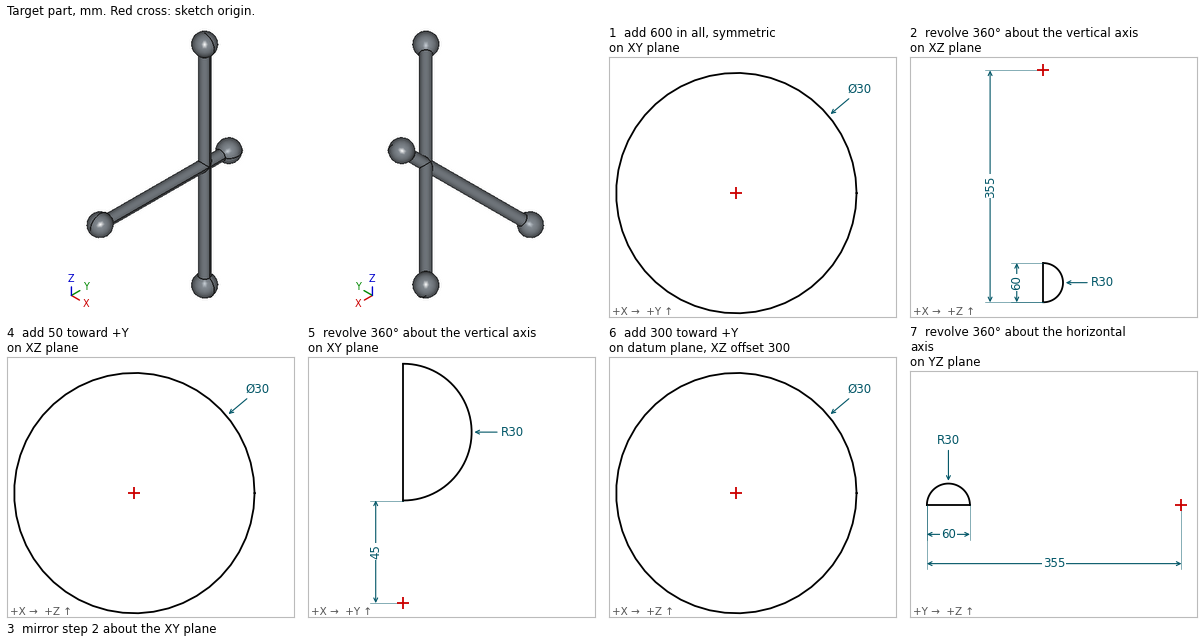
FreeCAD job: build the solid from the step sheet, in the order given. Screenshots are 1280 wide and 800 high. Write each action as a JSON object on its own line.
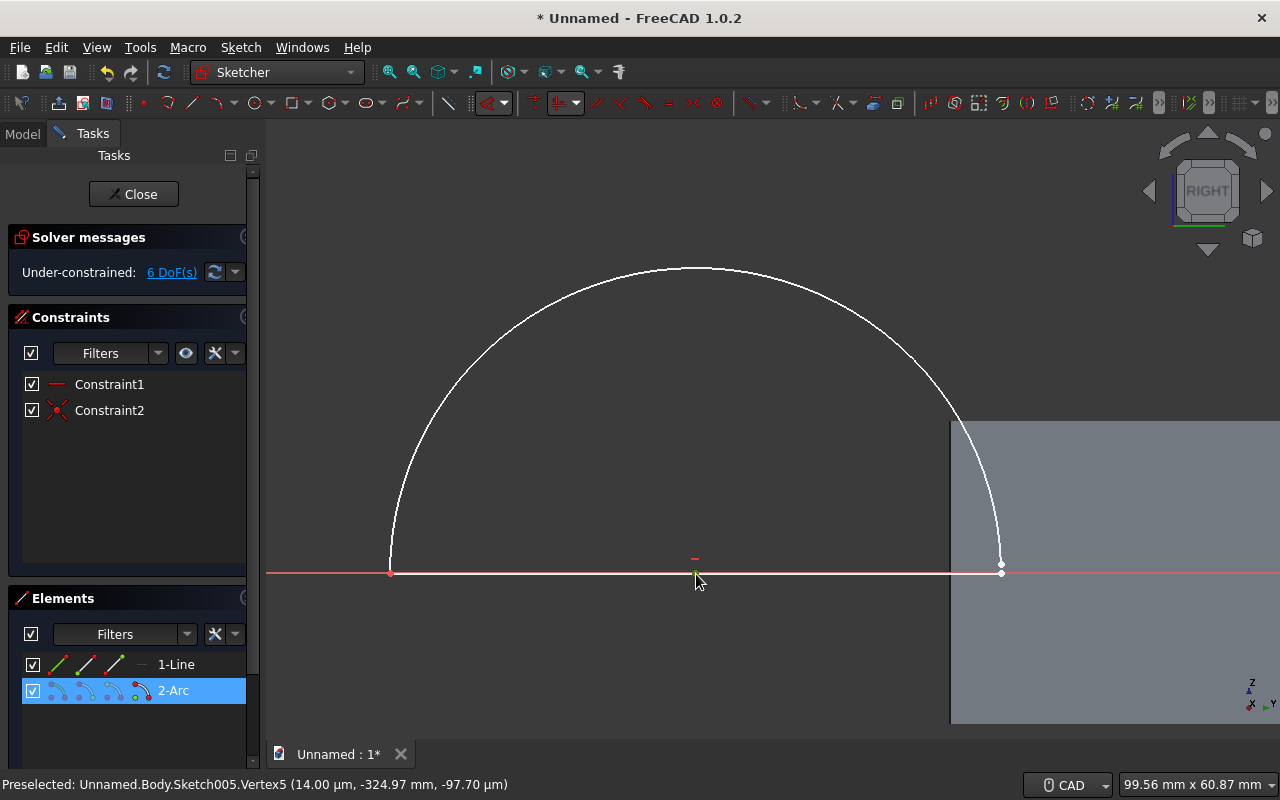
{"action": "left_click", "coordinate": [353, 573]}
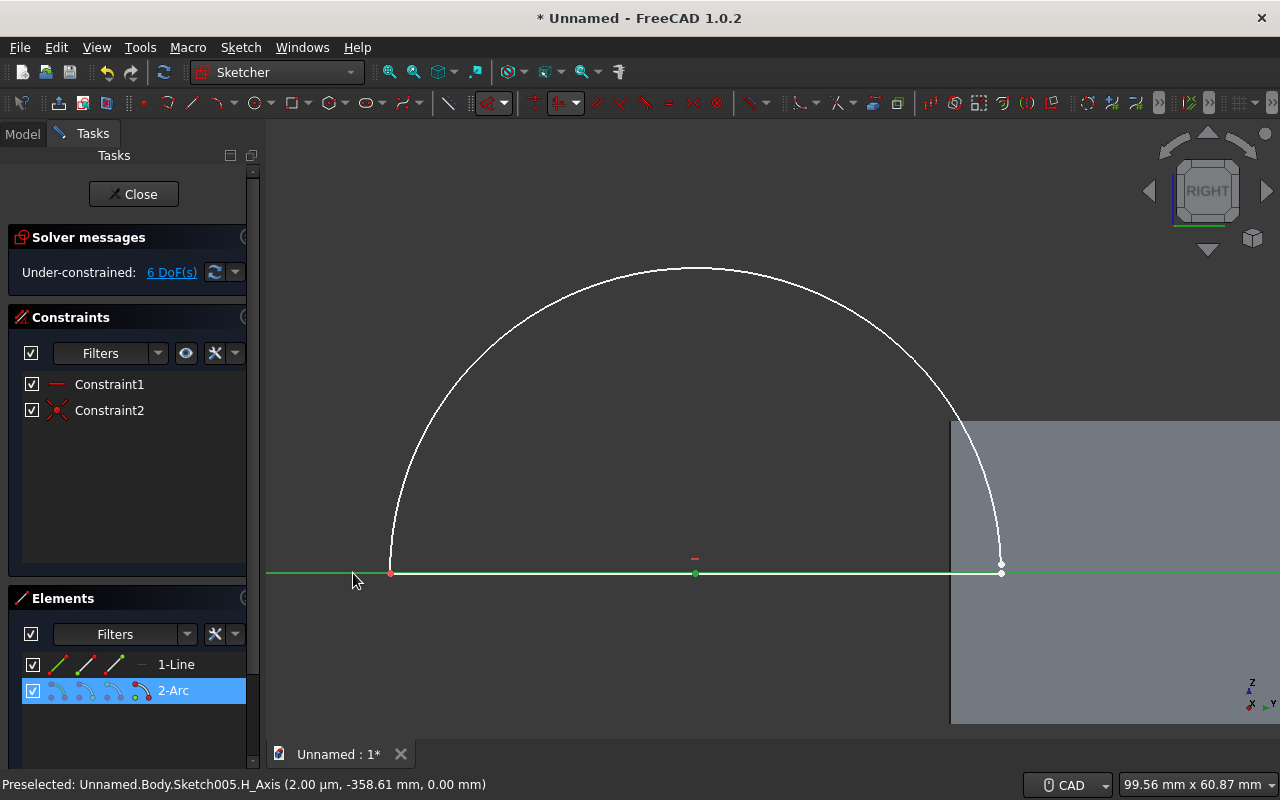
{"action": "left_click", "coordinate": [534, 104]}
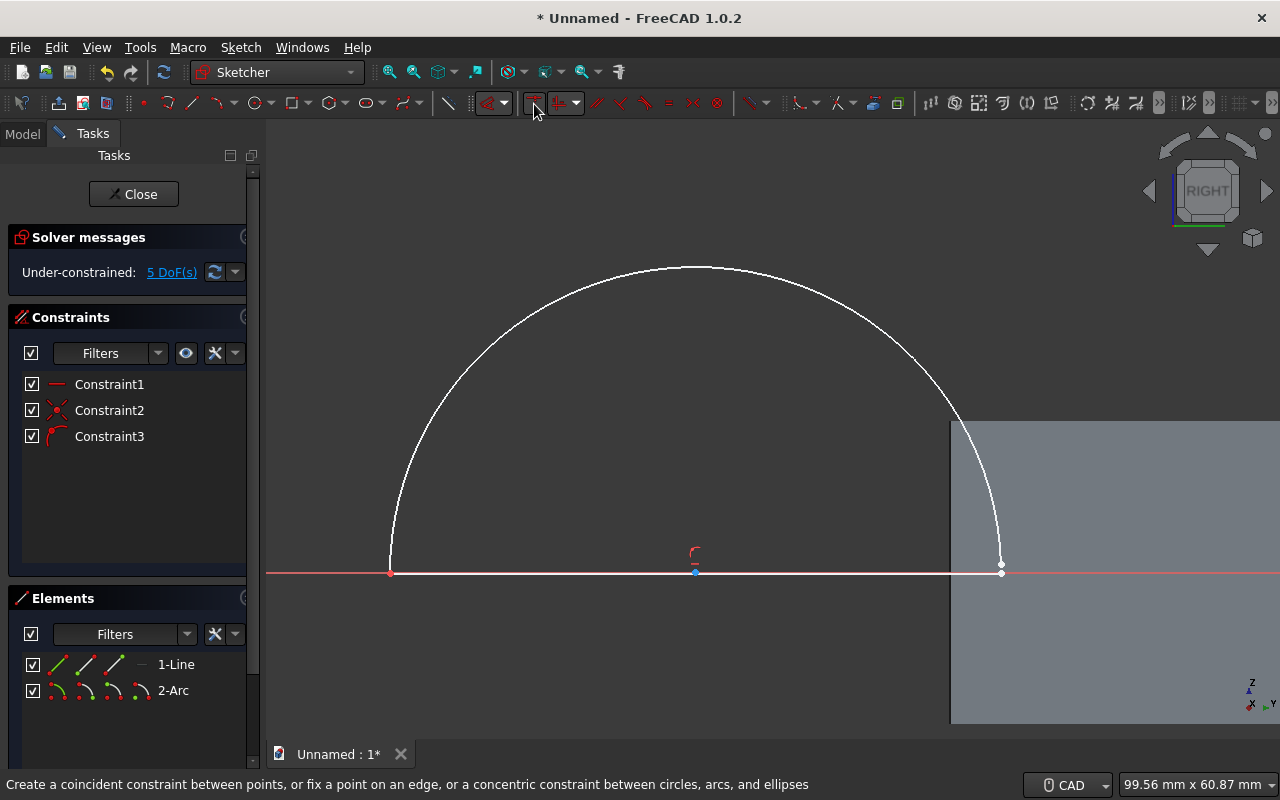
{"action": "left_click", "coordinate": [870, 322]}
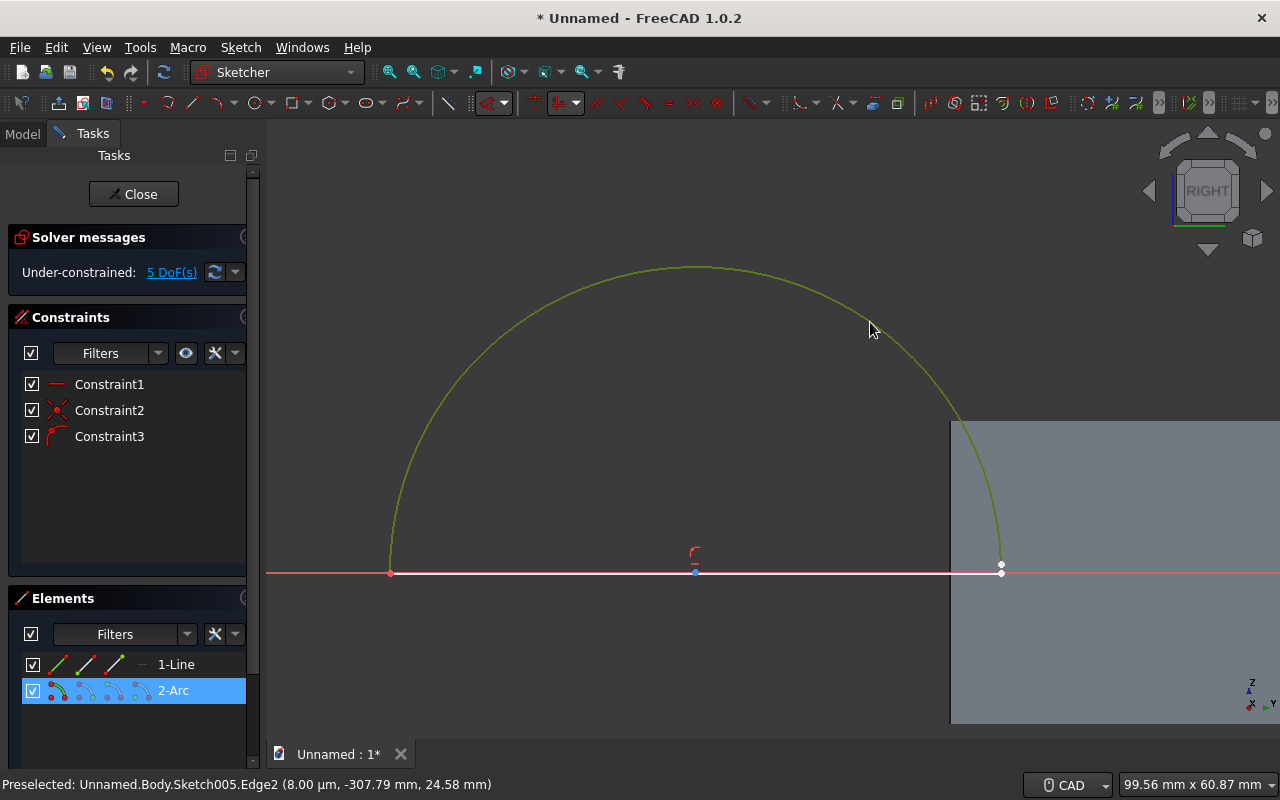
{"action": "key", "text": "k r"}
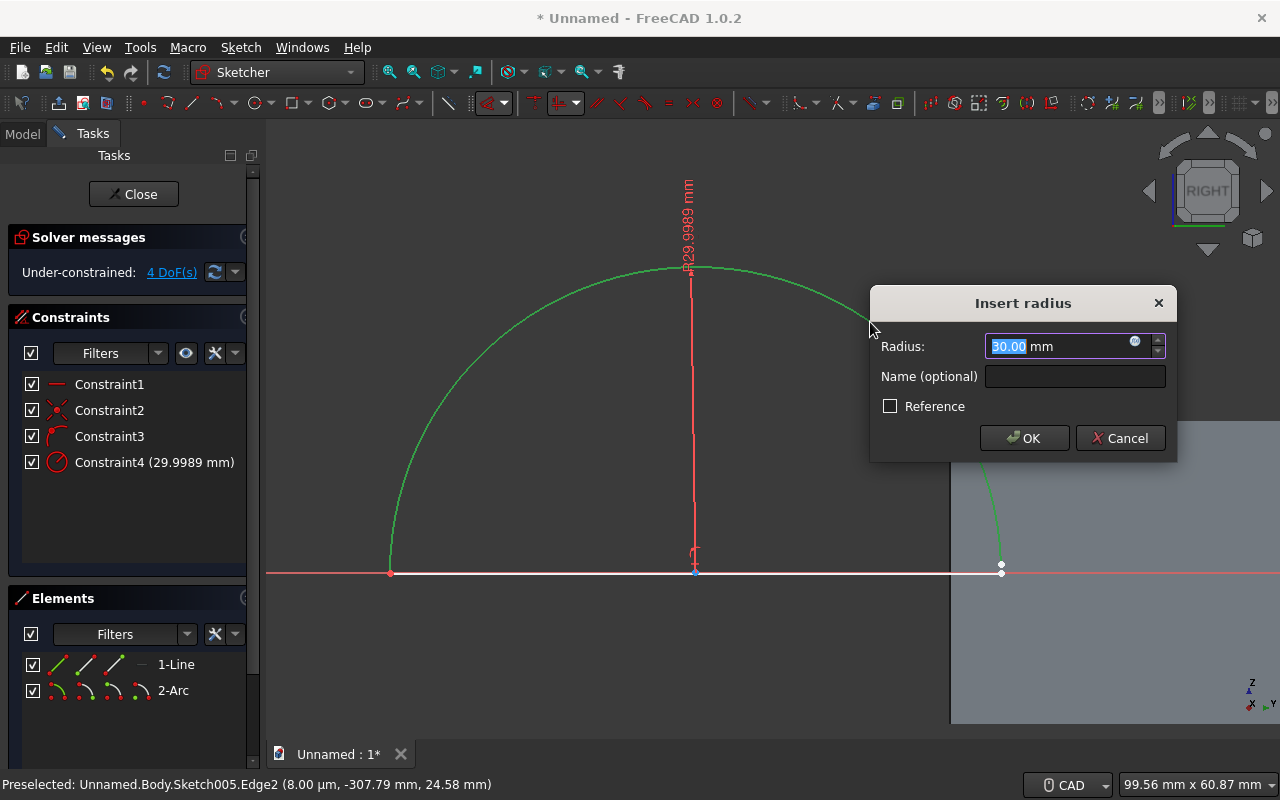
{"action": "type", "text": "30"}
{"action": "key", "text": "Return"}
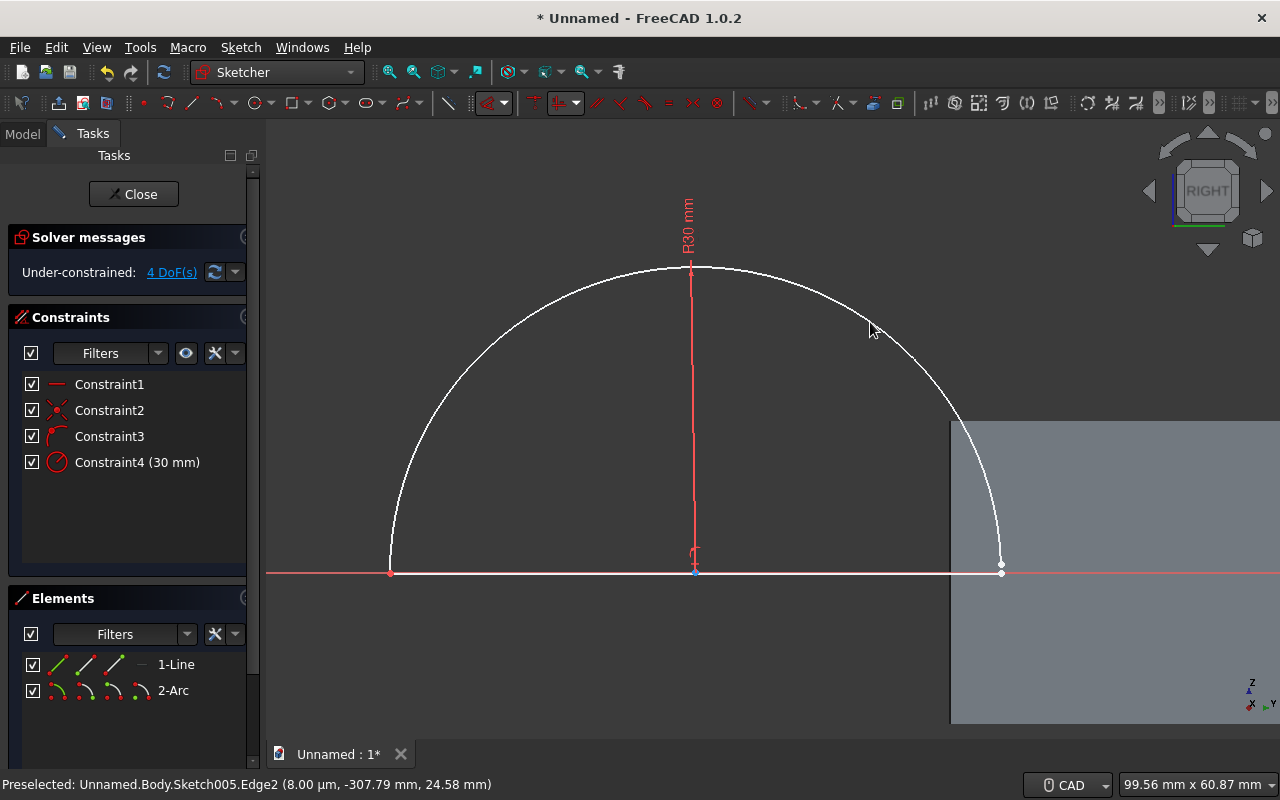
{"action": "left_click", "coordinate": [390, 574]}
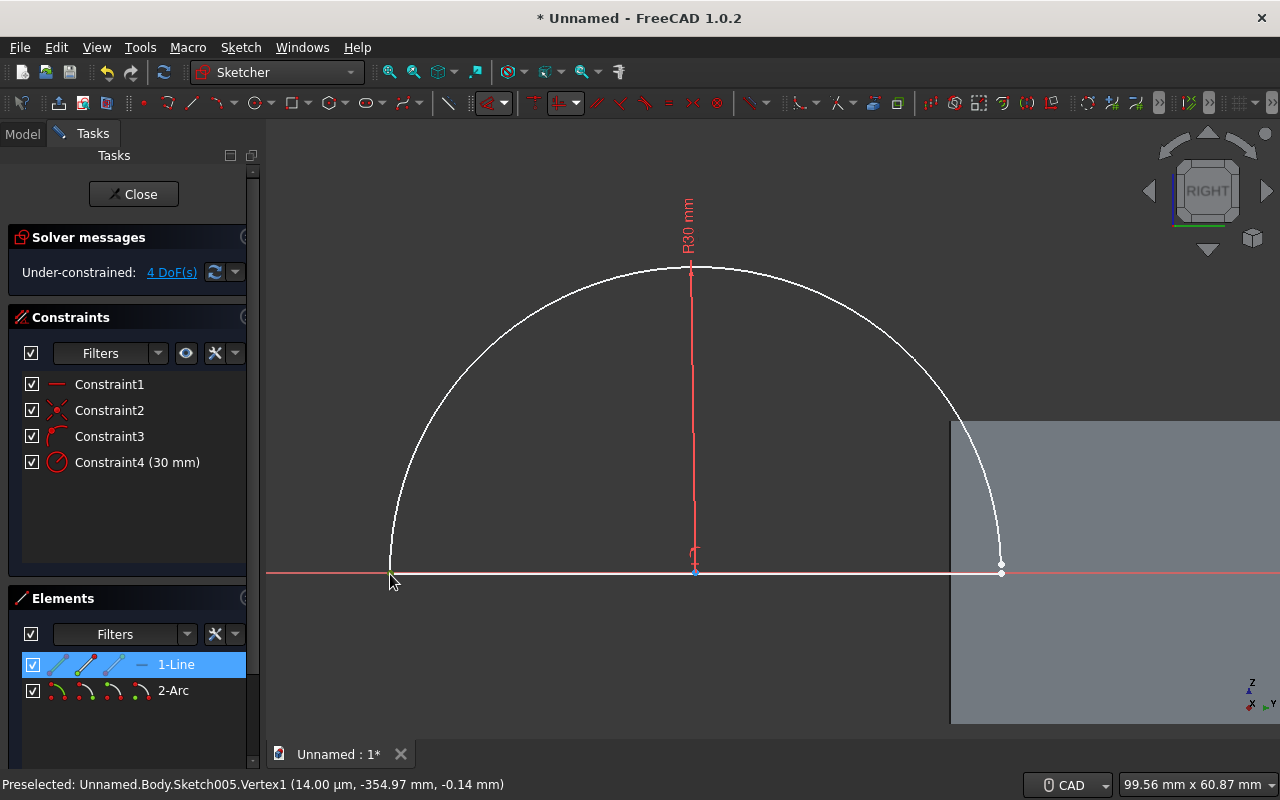
{"action": "left_click", "coordinate": [353, 573]}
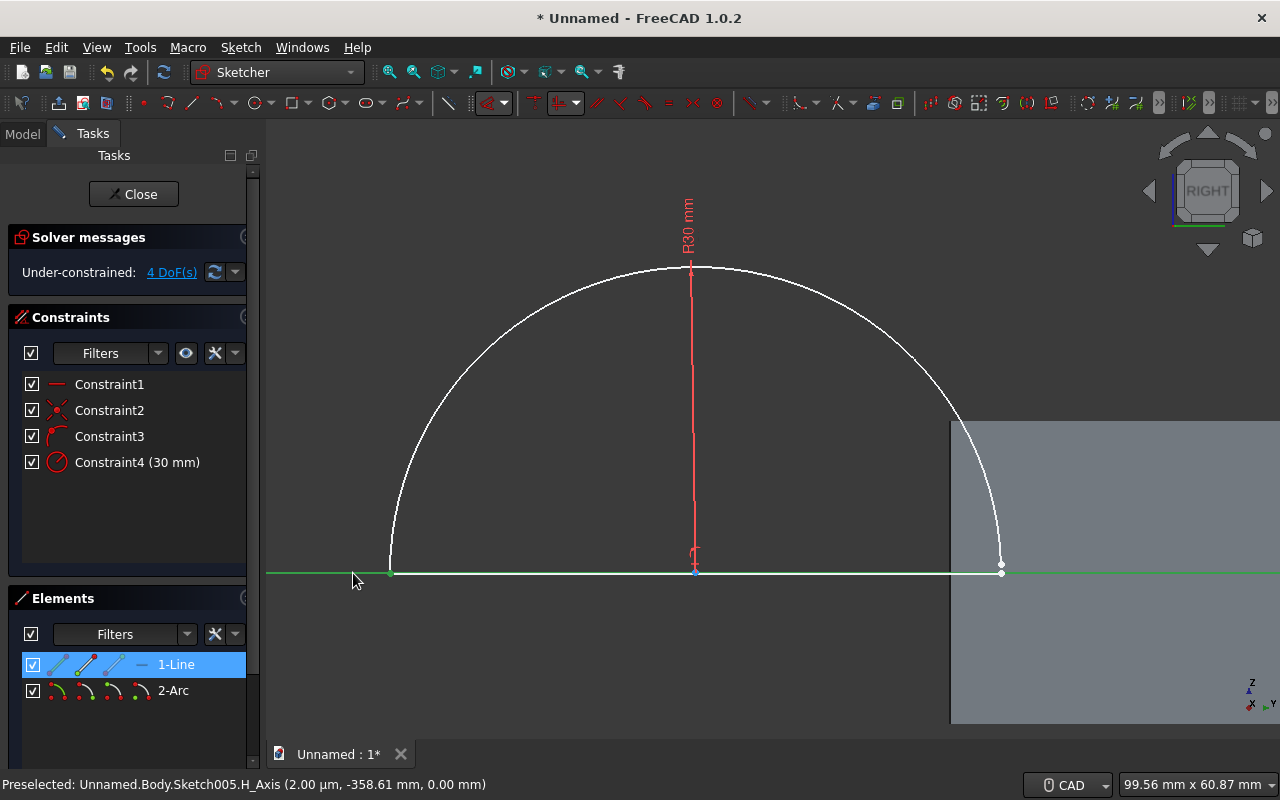
{"action": "left_click", "coordinate": [534, 104]}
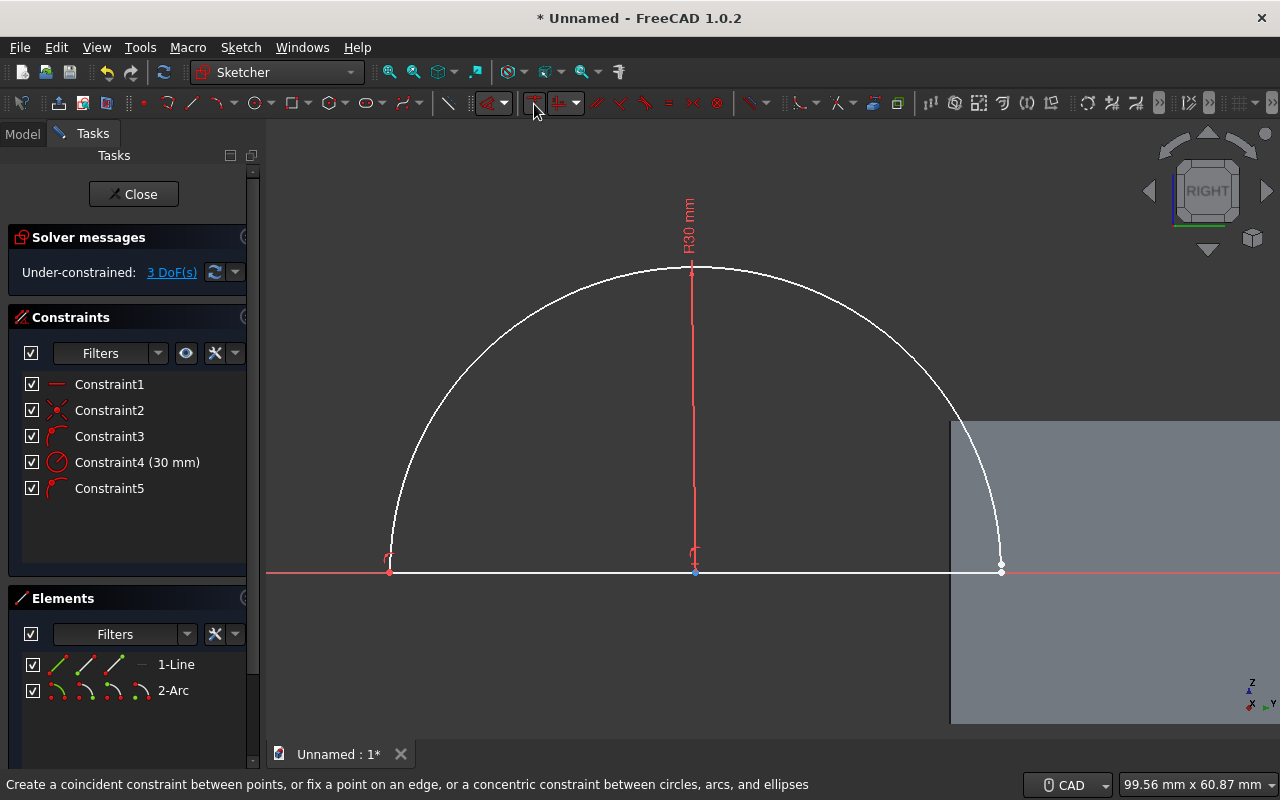
{"action": "left_click", "coordinate": [1001, 565]}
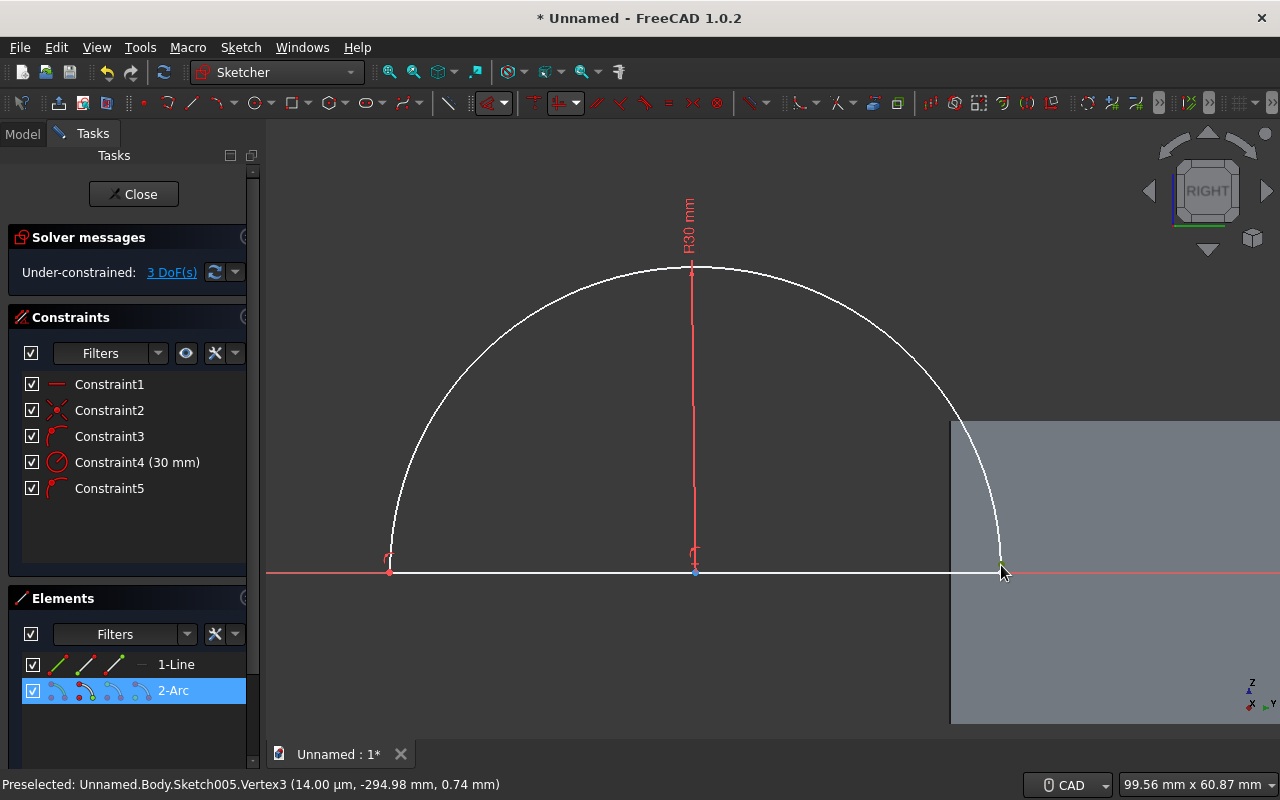
{"action": "left_click", "coordinate": [353, 573]}